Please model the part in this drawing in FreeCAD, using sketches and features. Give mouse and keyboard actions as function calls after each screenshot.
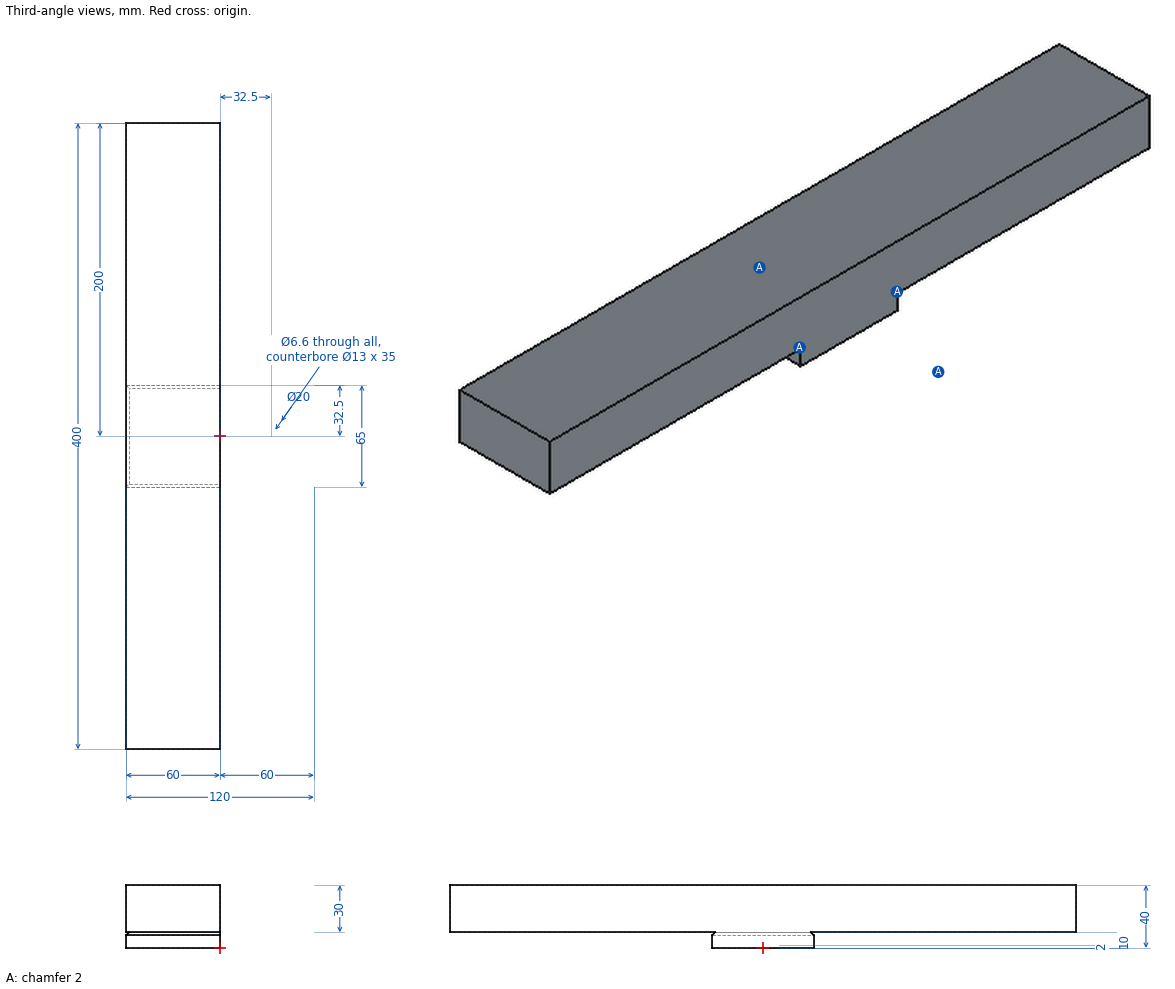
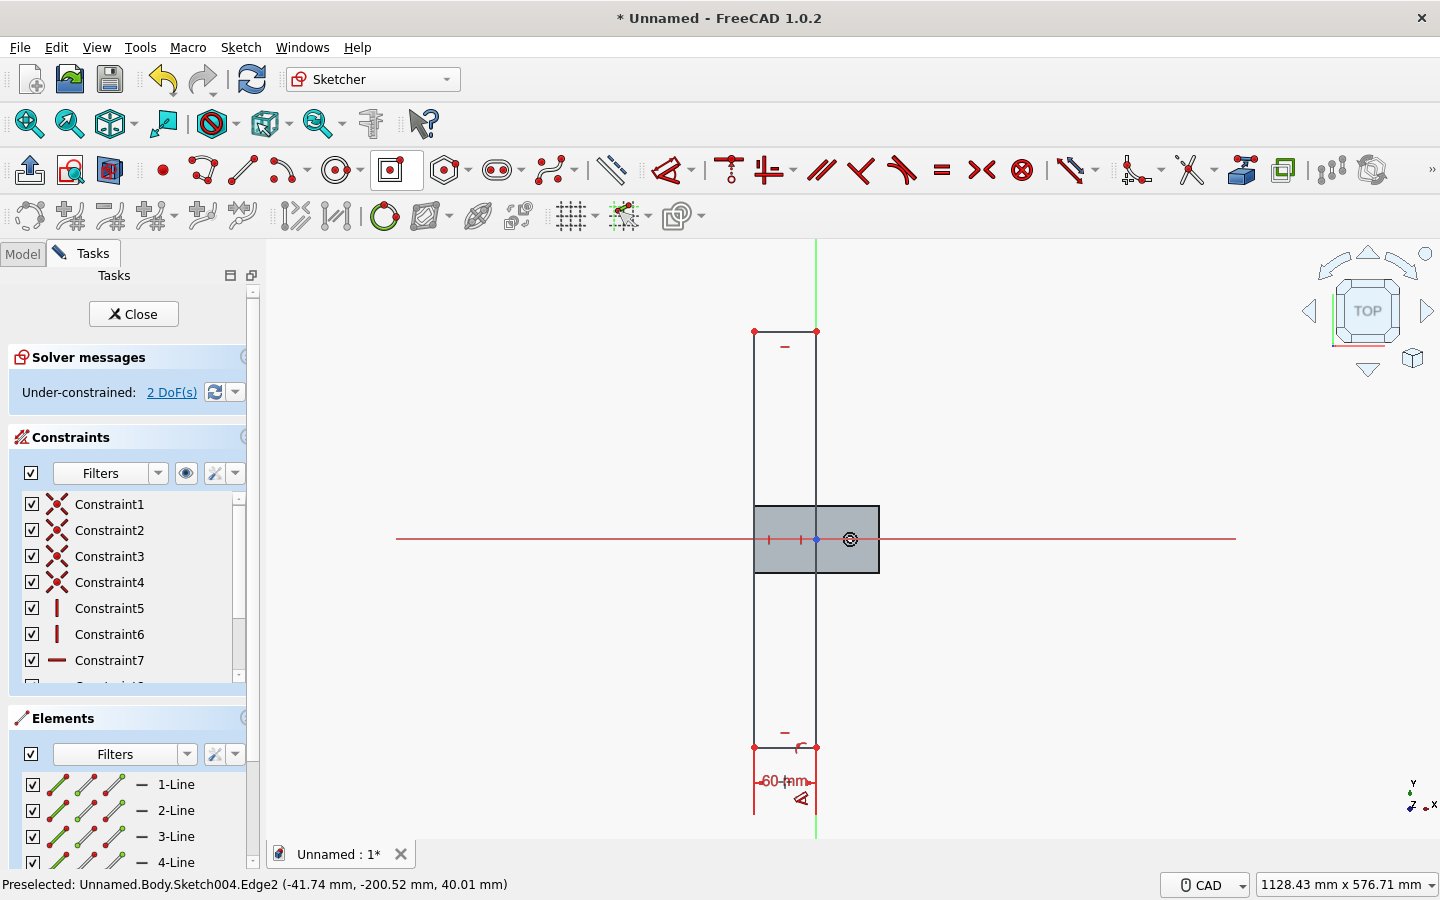
click(754, 457)
click(720, 444)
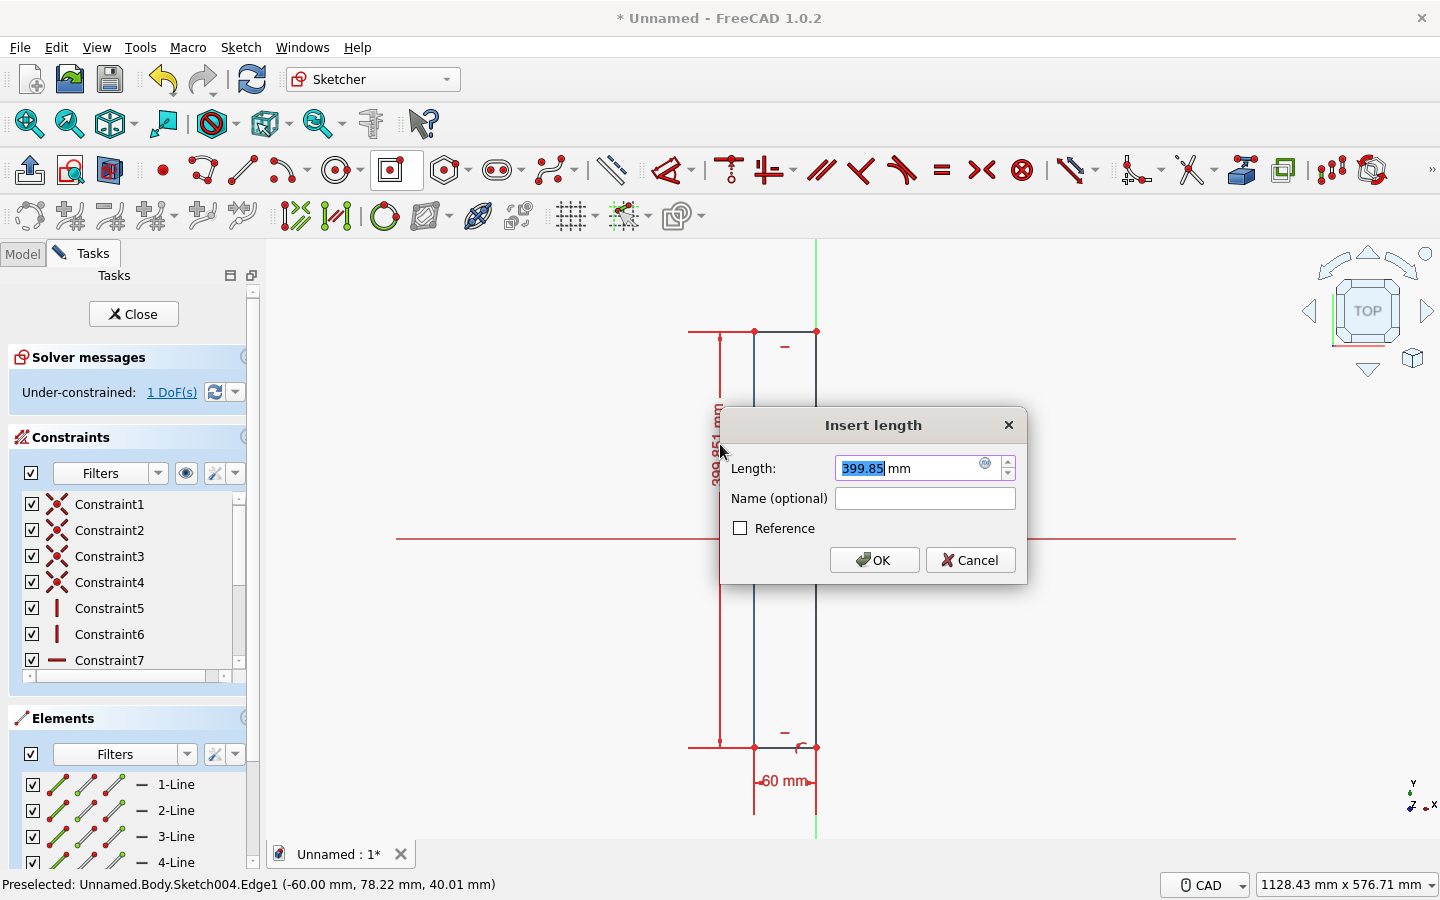
text(400)
key(Return)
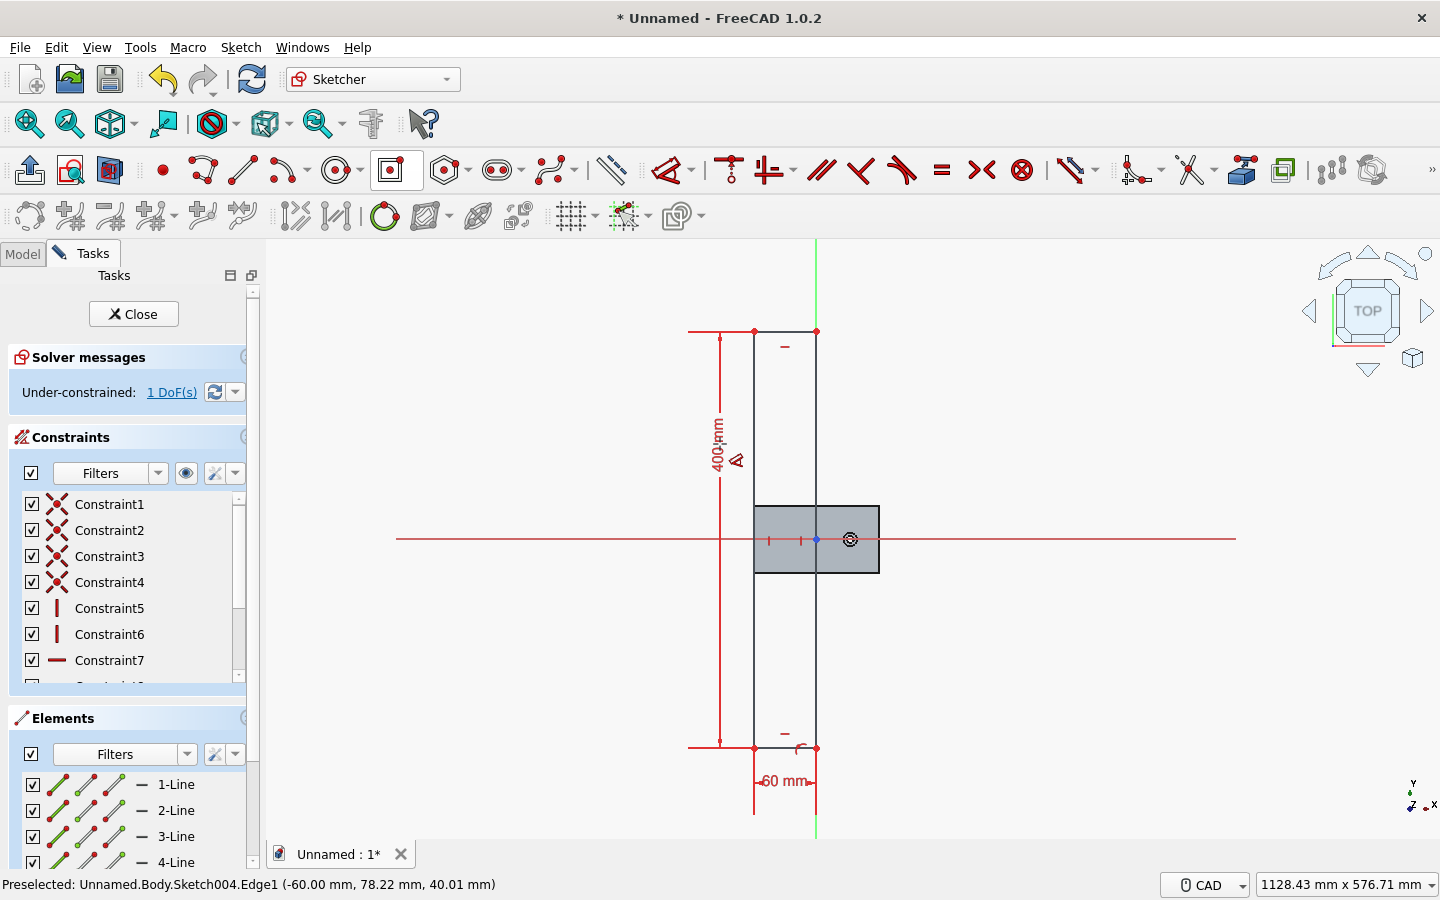
click(754, 332)
click(850, 436)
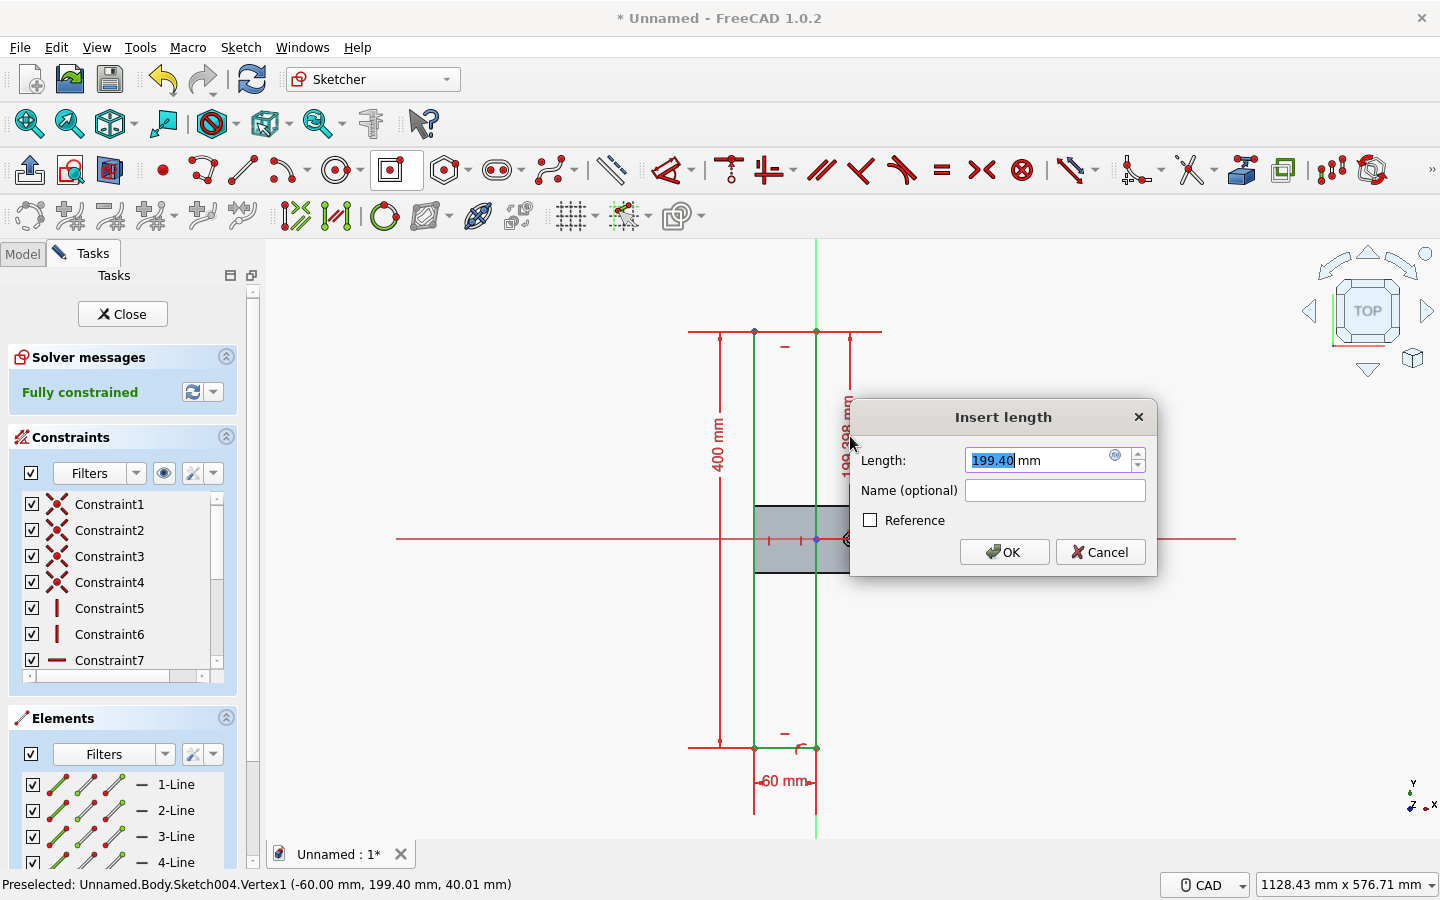
text(200)
key(Return)
key(Escape)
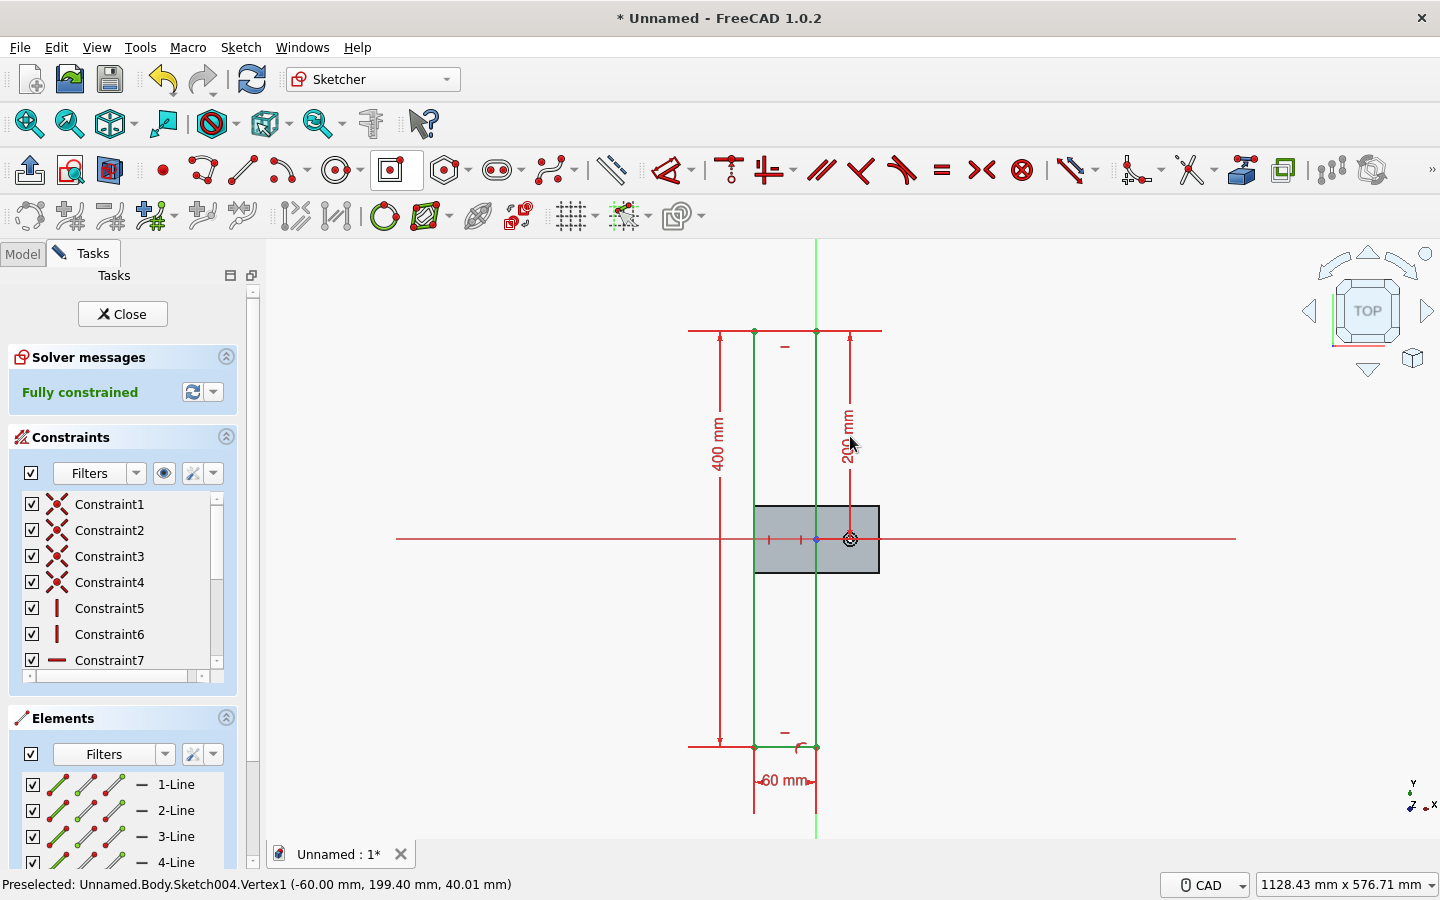
click(123, 314)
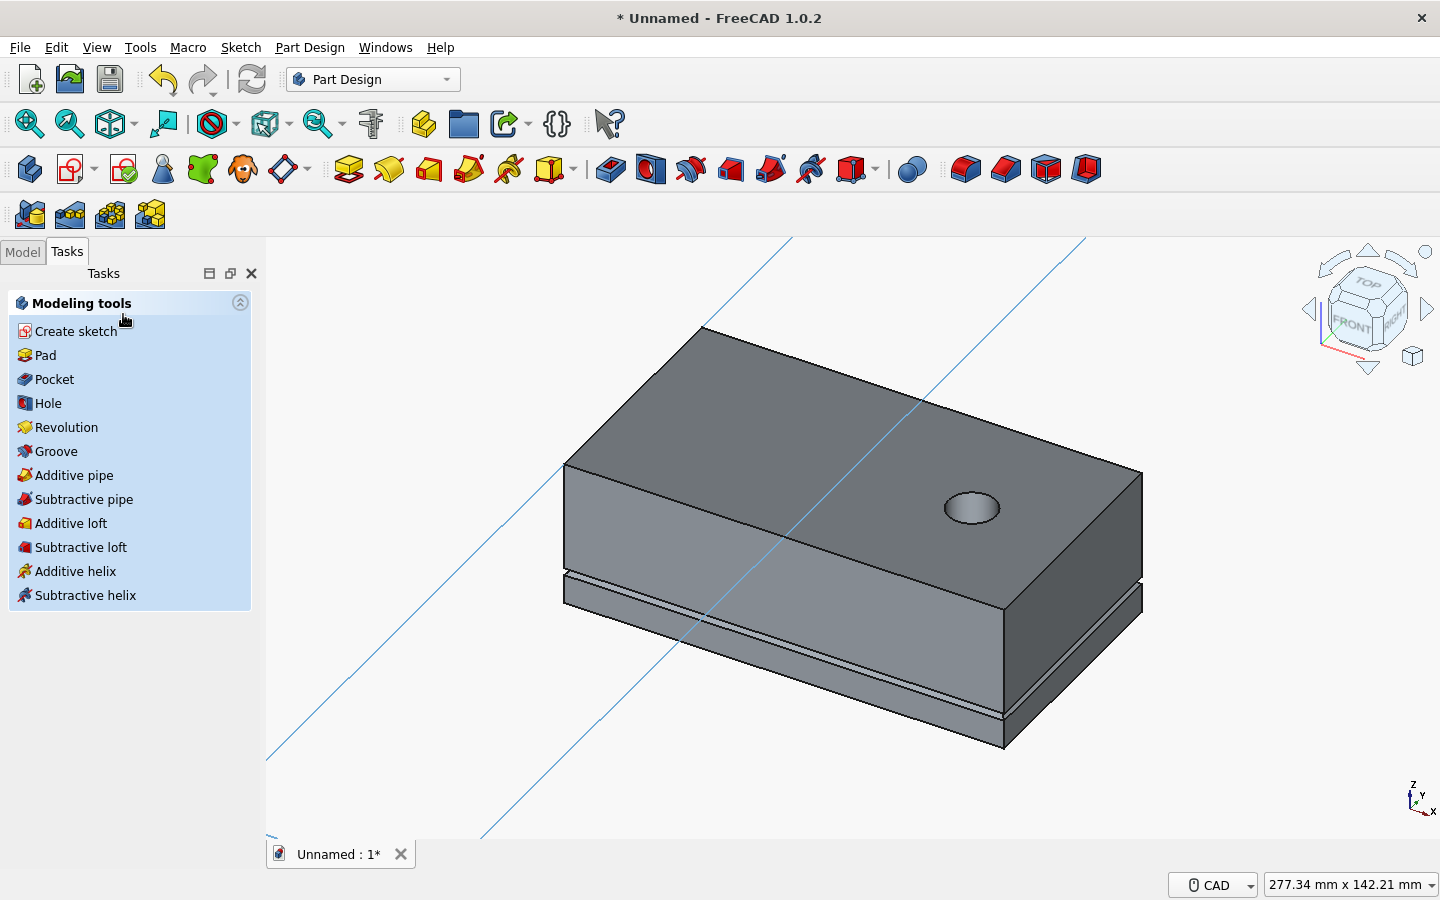
click(350, 170)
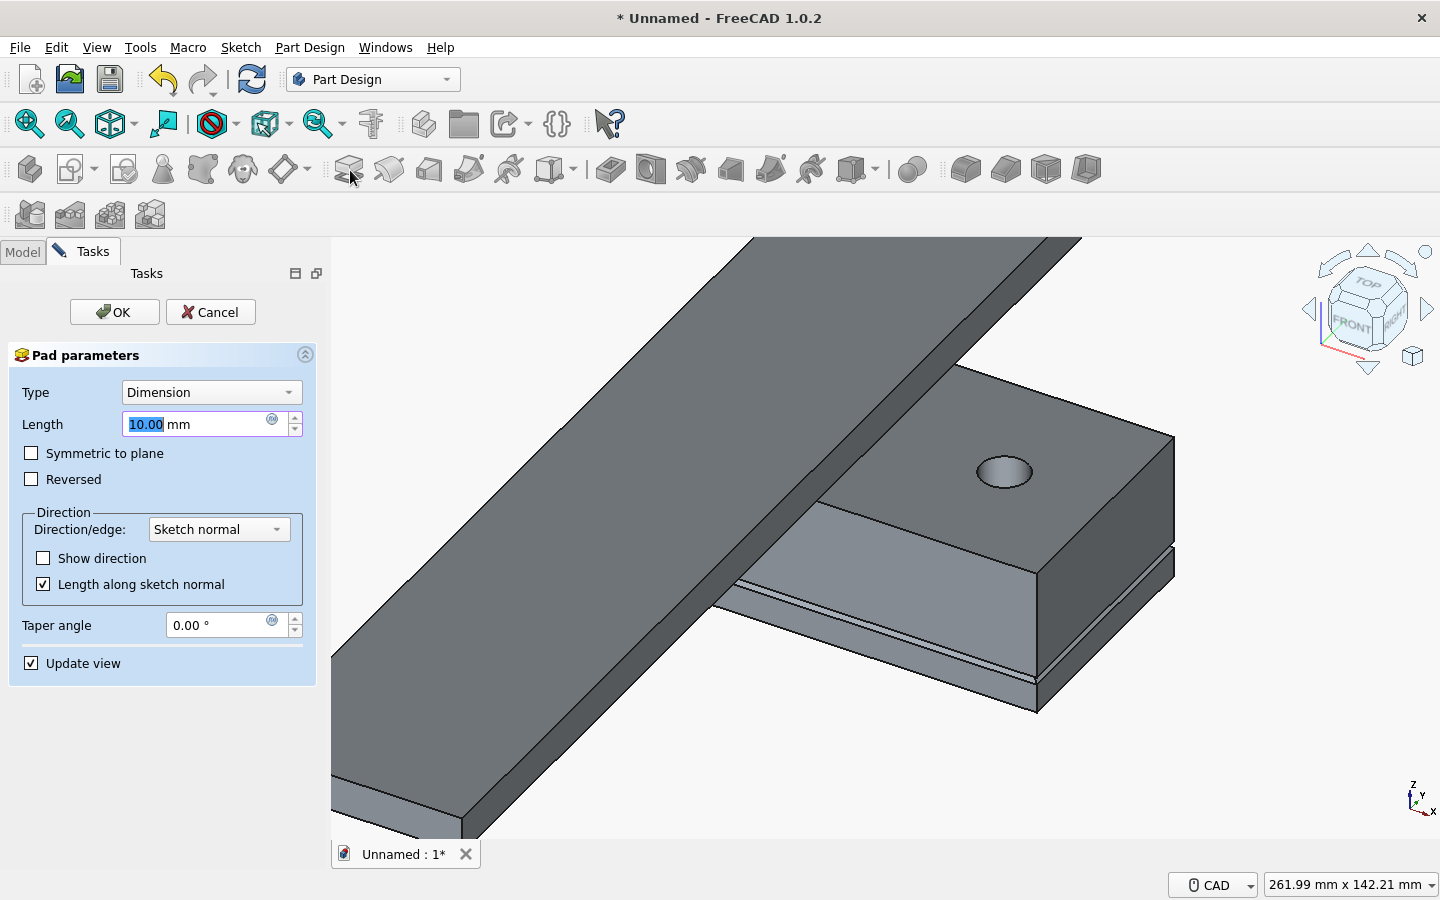
text(30)
key(Tab)